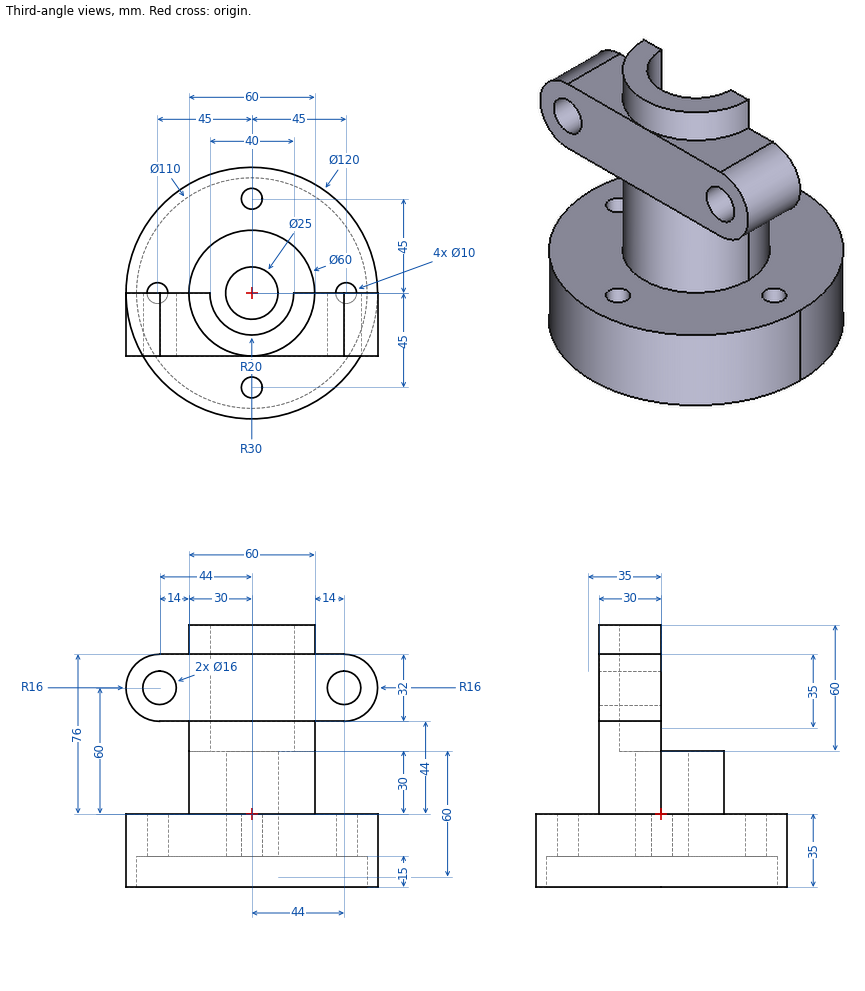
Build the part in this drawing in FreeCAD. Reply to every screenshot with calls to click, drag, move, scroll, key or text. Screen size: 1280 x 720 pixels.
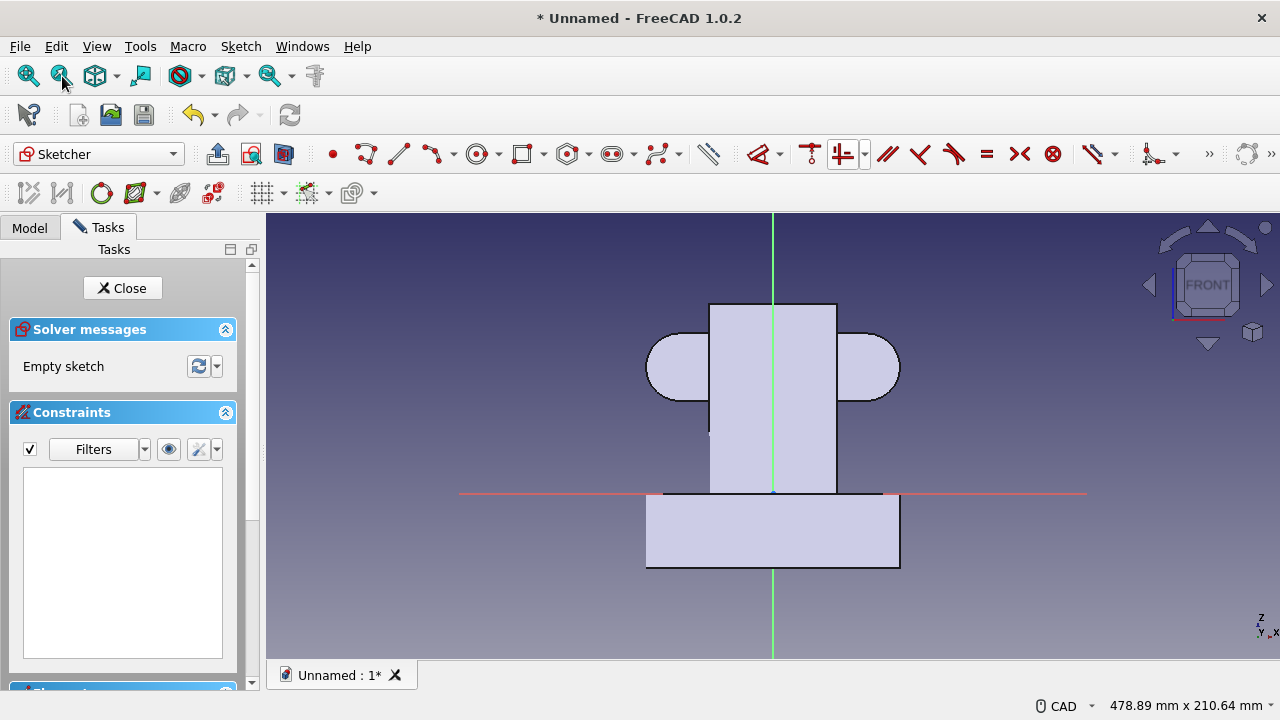
click(284, 154)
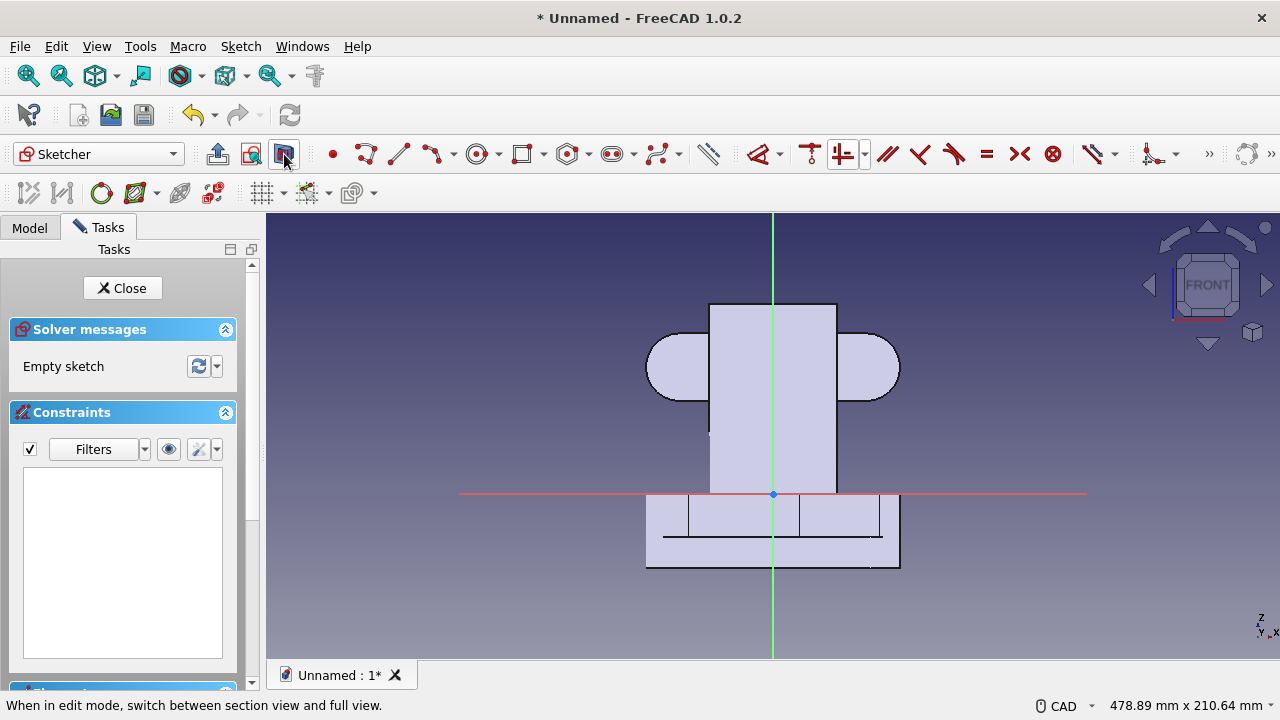
scroll(856, 387, up, 3)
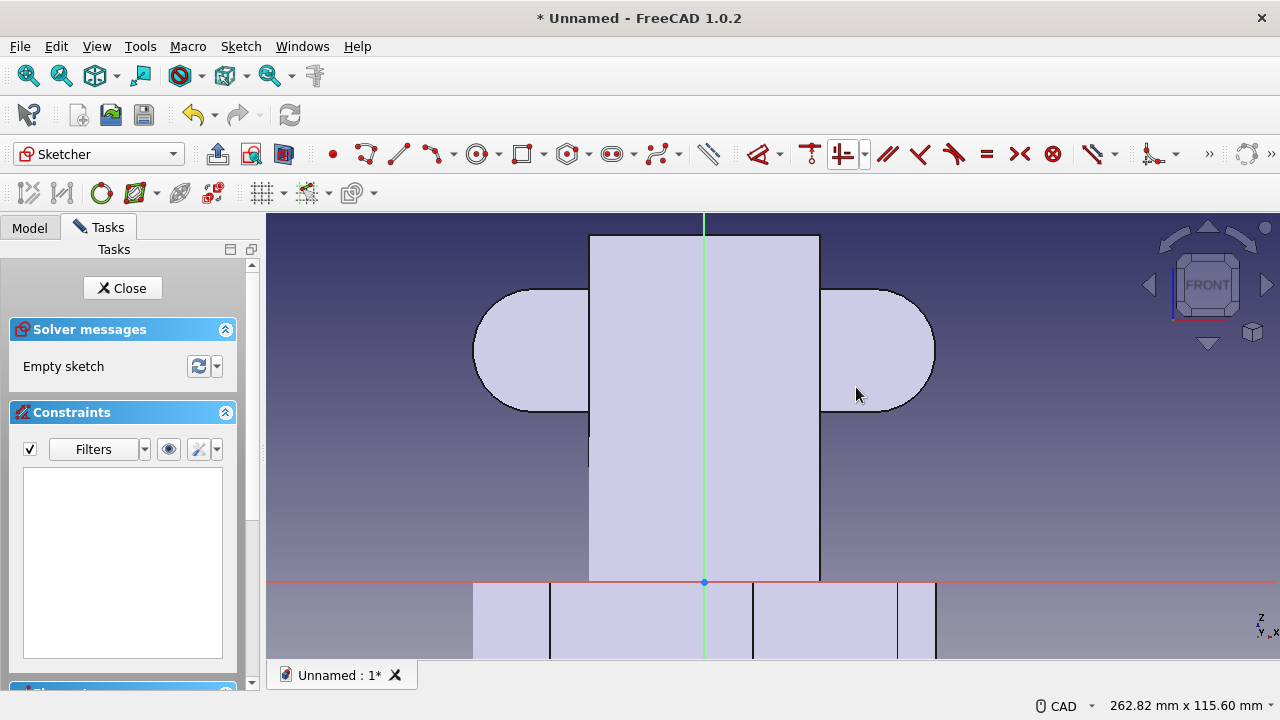
click(522, 154)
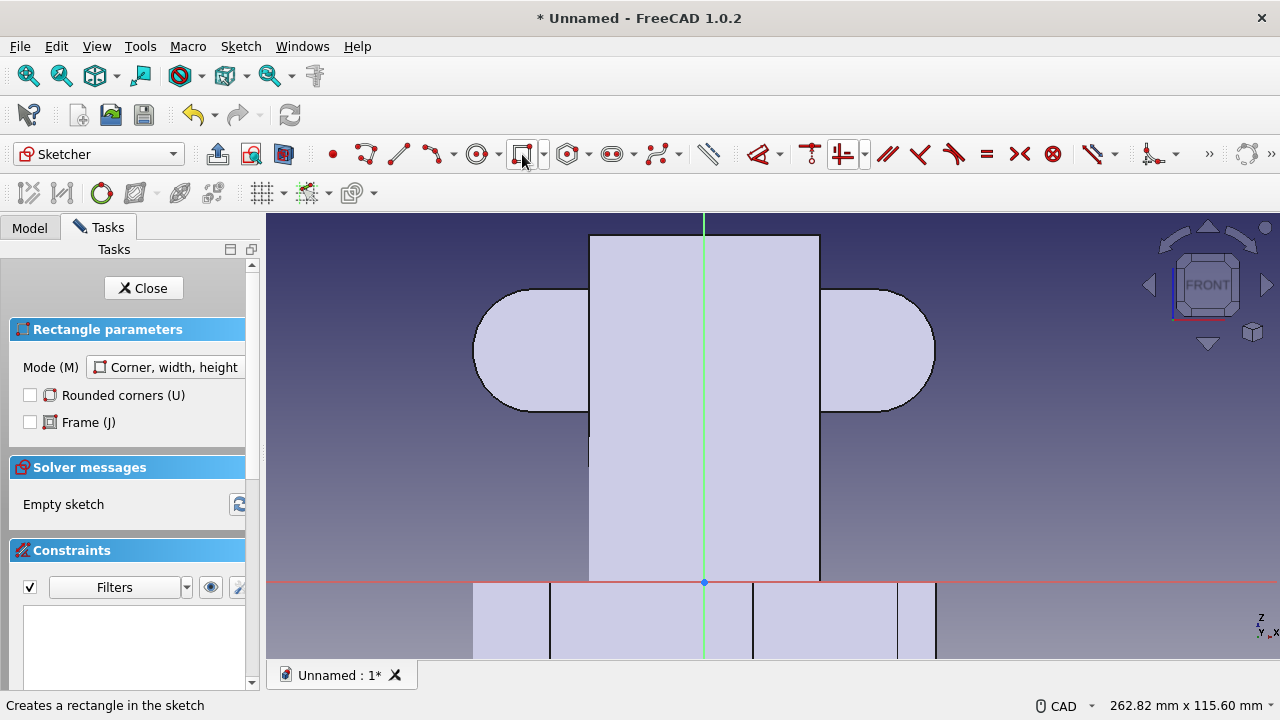
click(589, 289)
move(820, 412)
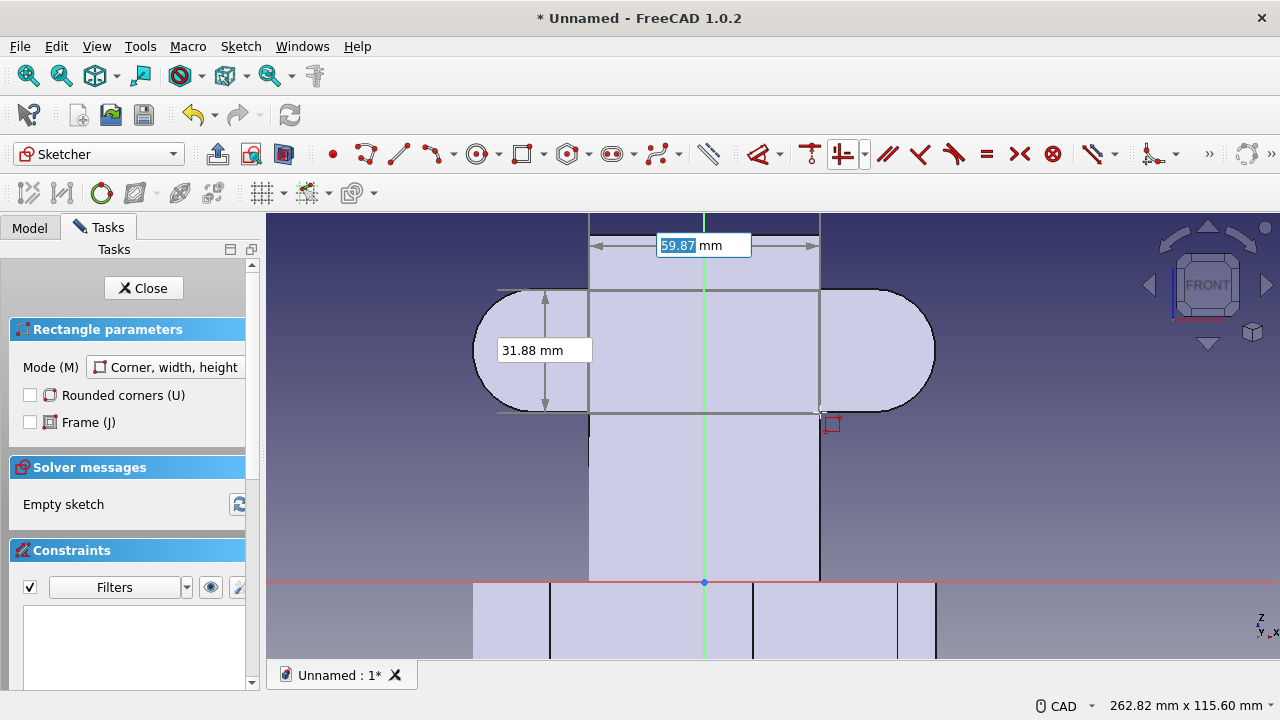
text(60)
key(Tab)
text(32)
key(Return)
key(Escape)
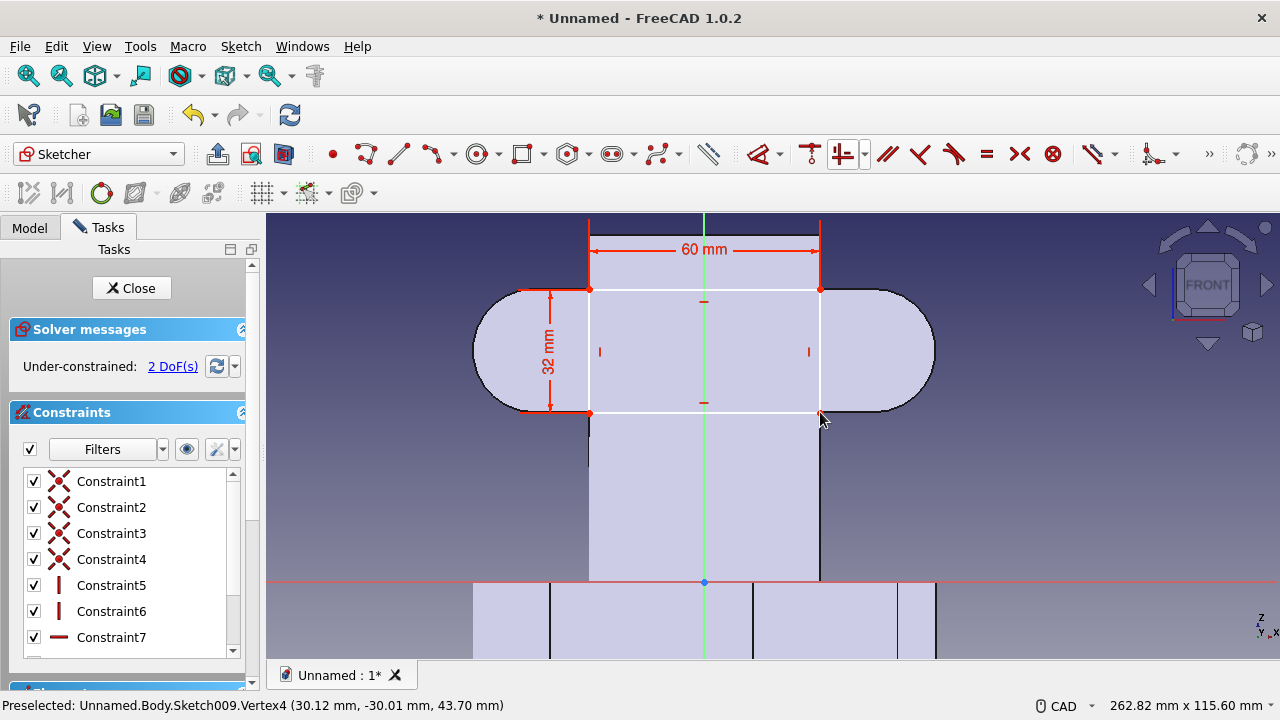
click(758, 154)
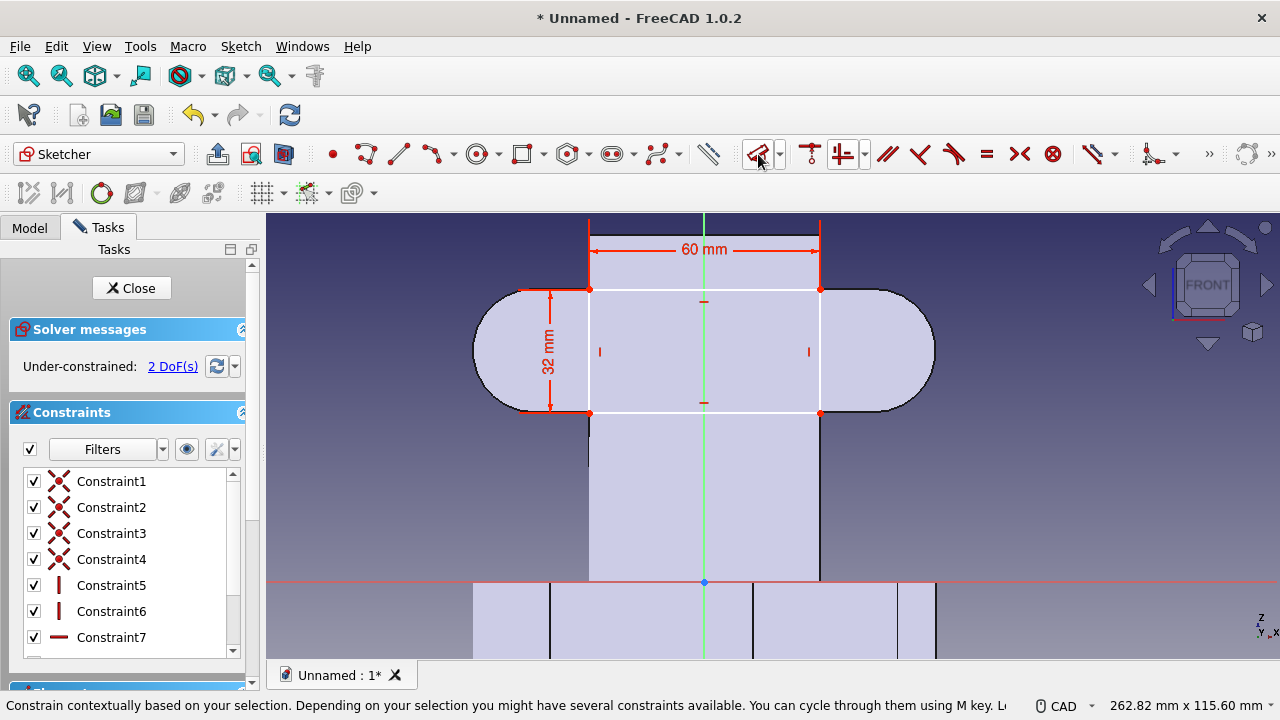
click(589, 290)
click(647, 616)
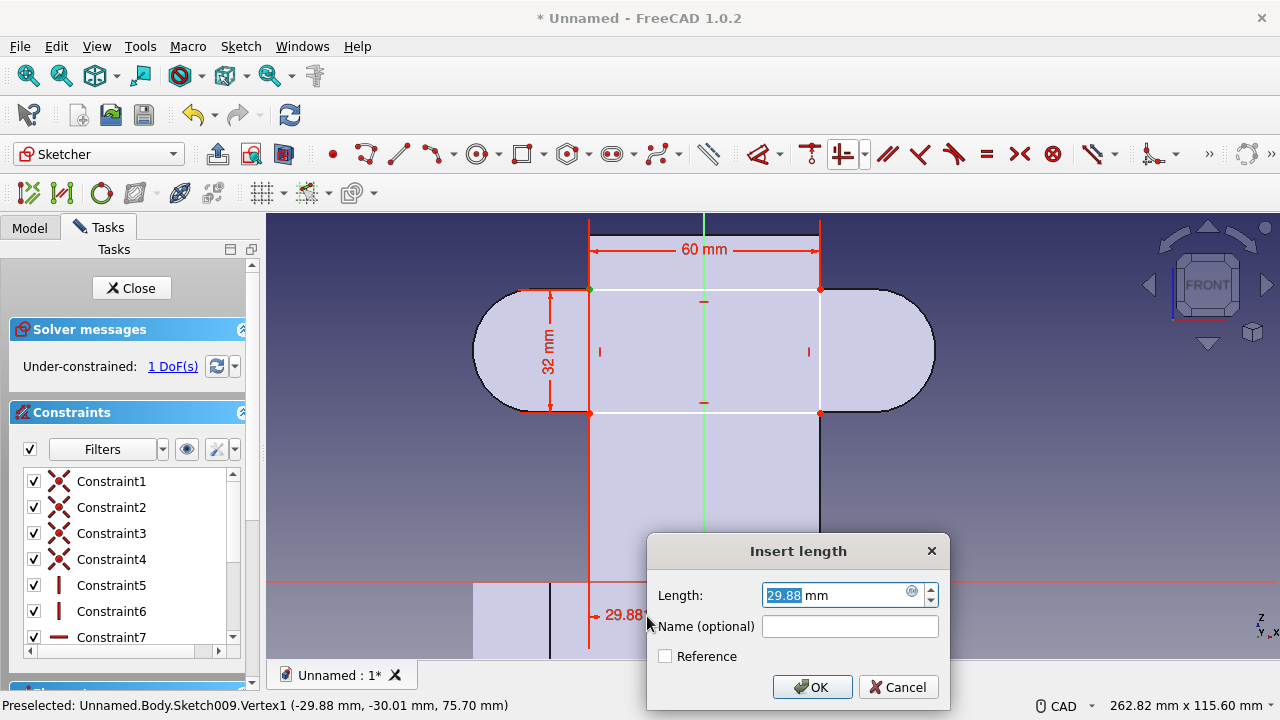
text(30)
key(Return)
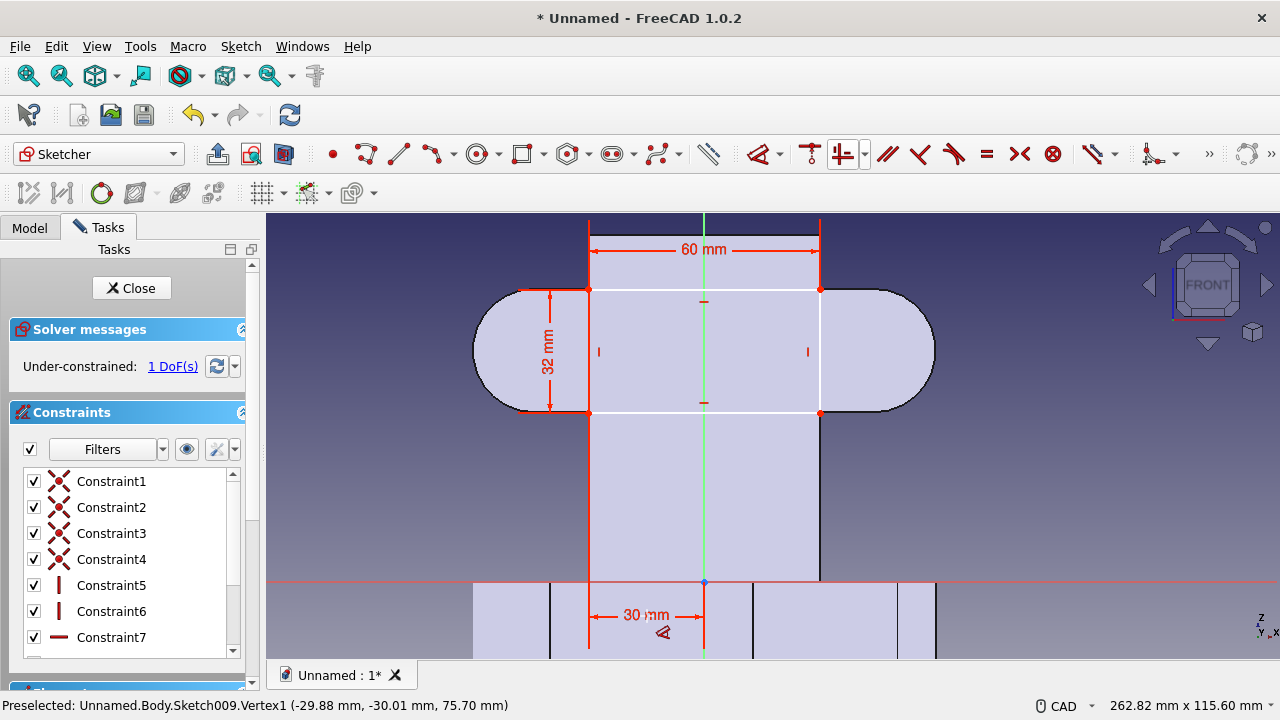
click(589, 290)
click(555, 436)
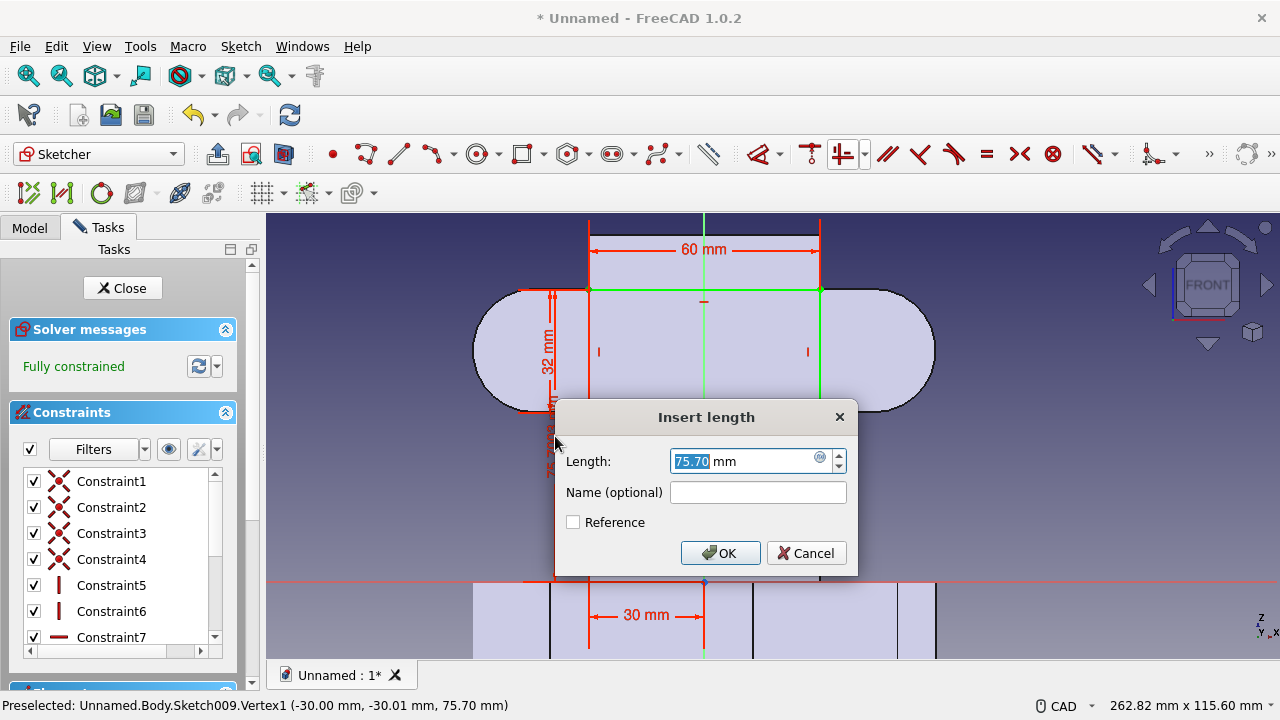
text(76)
key(Return)
key(Escape)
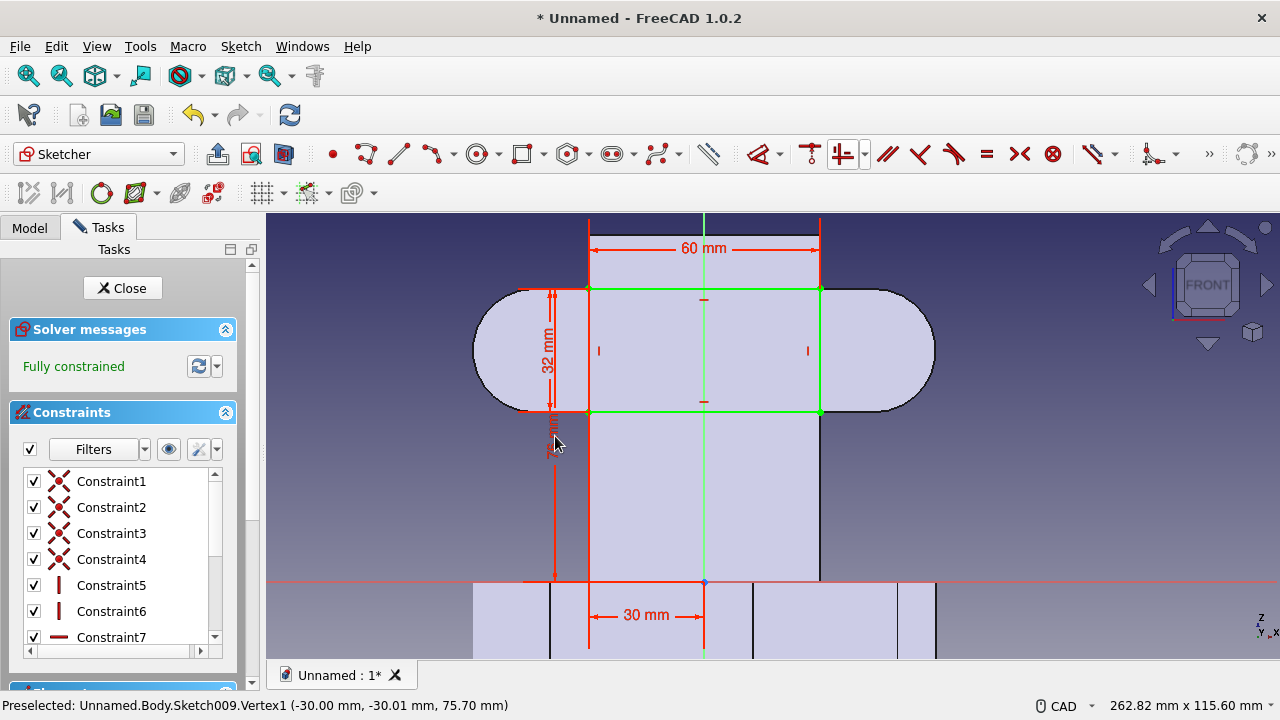
click(123, 288)